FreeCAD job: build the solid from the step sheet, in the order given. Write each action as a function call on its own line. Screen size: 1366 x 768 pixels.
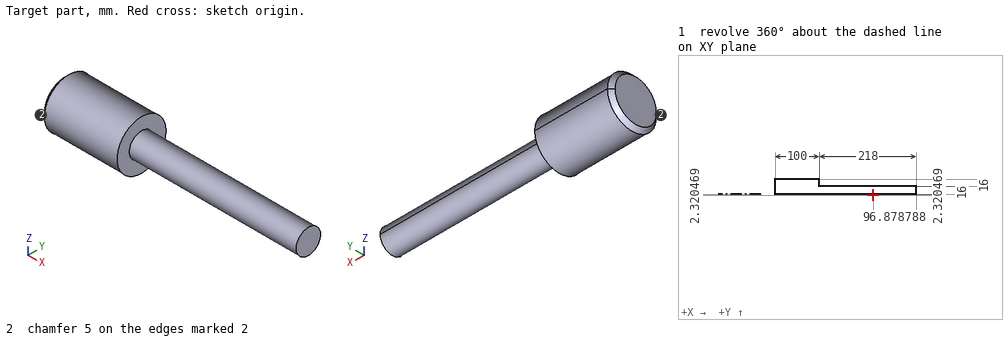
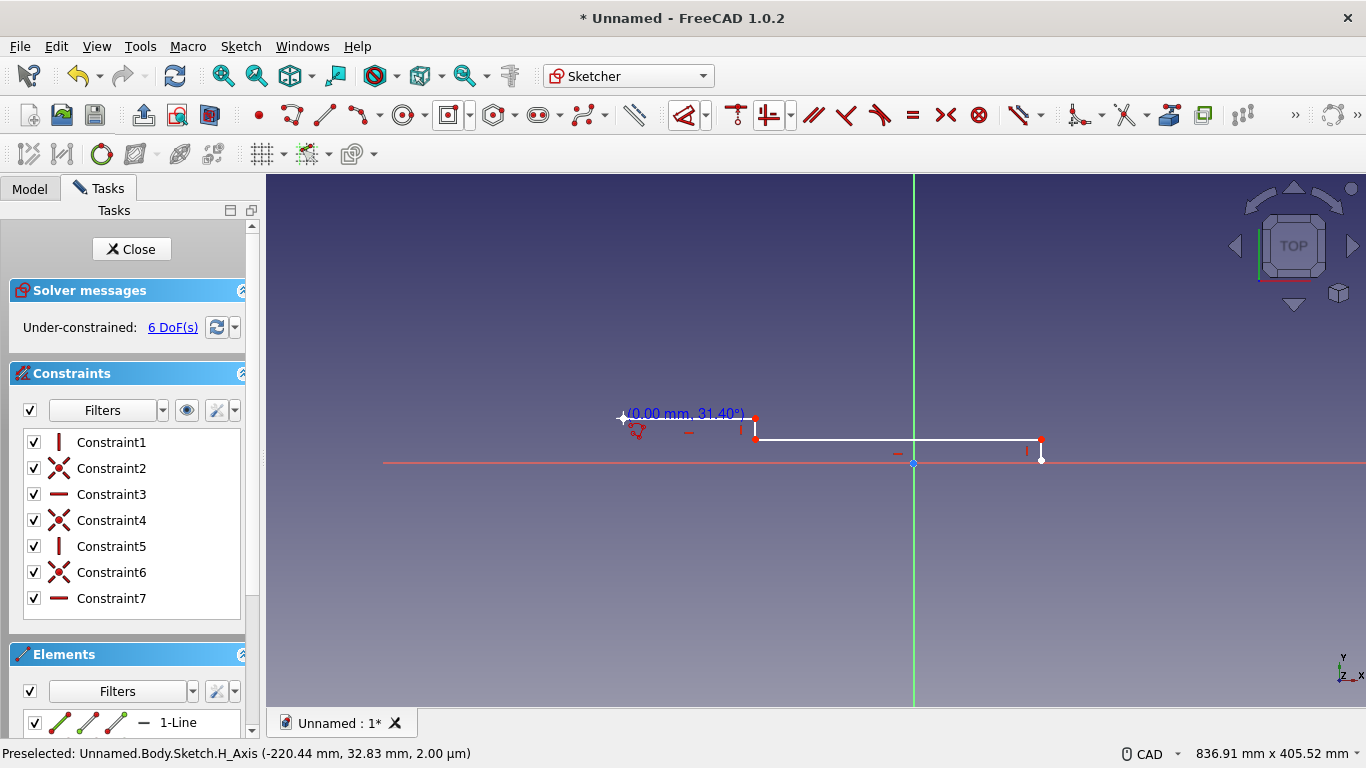
scroll(623, 460, up, 9)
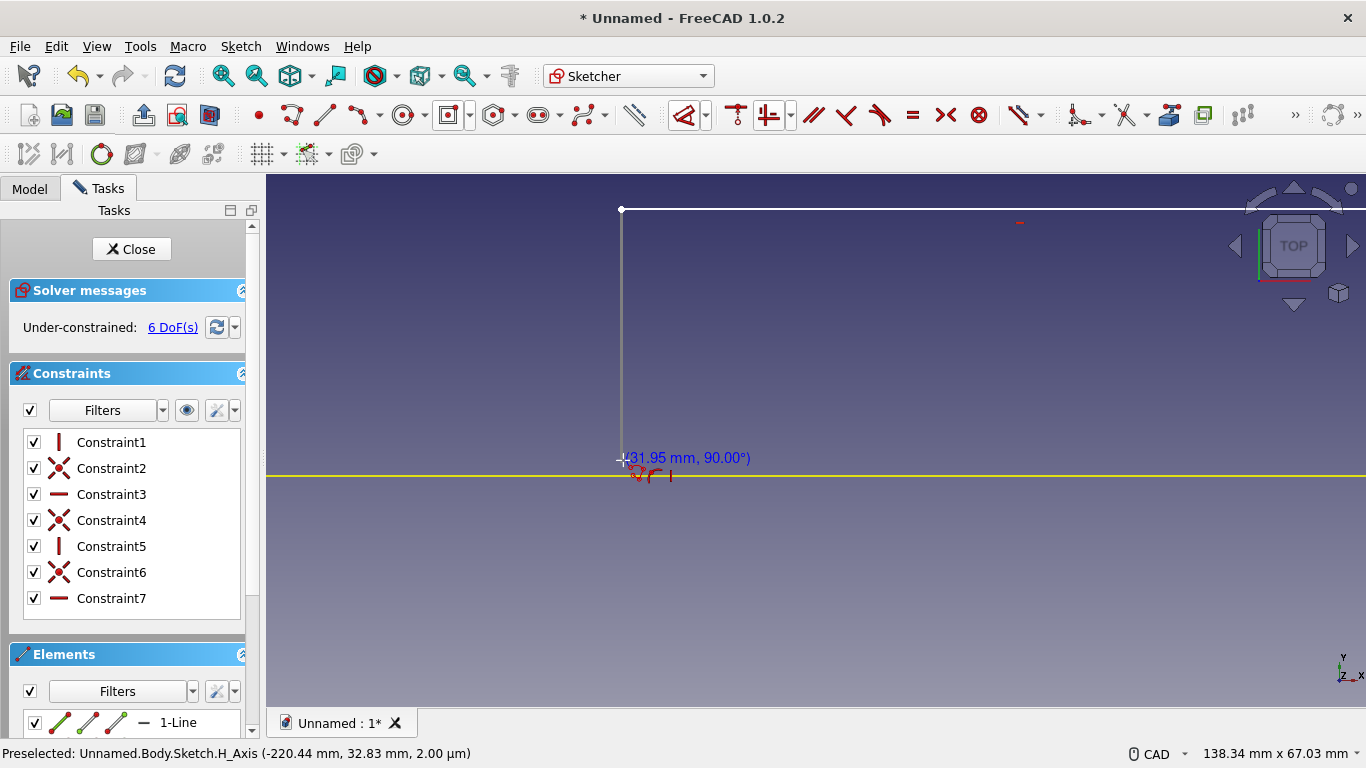
click(621, 458)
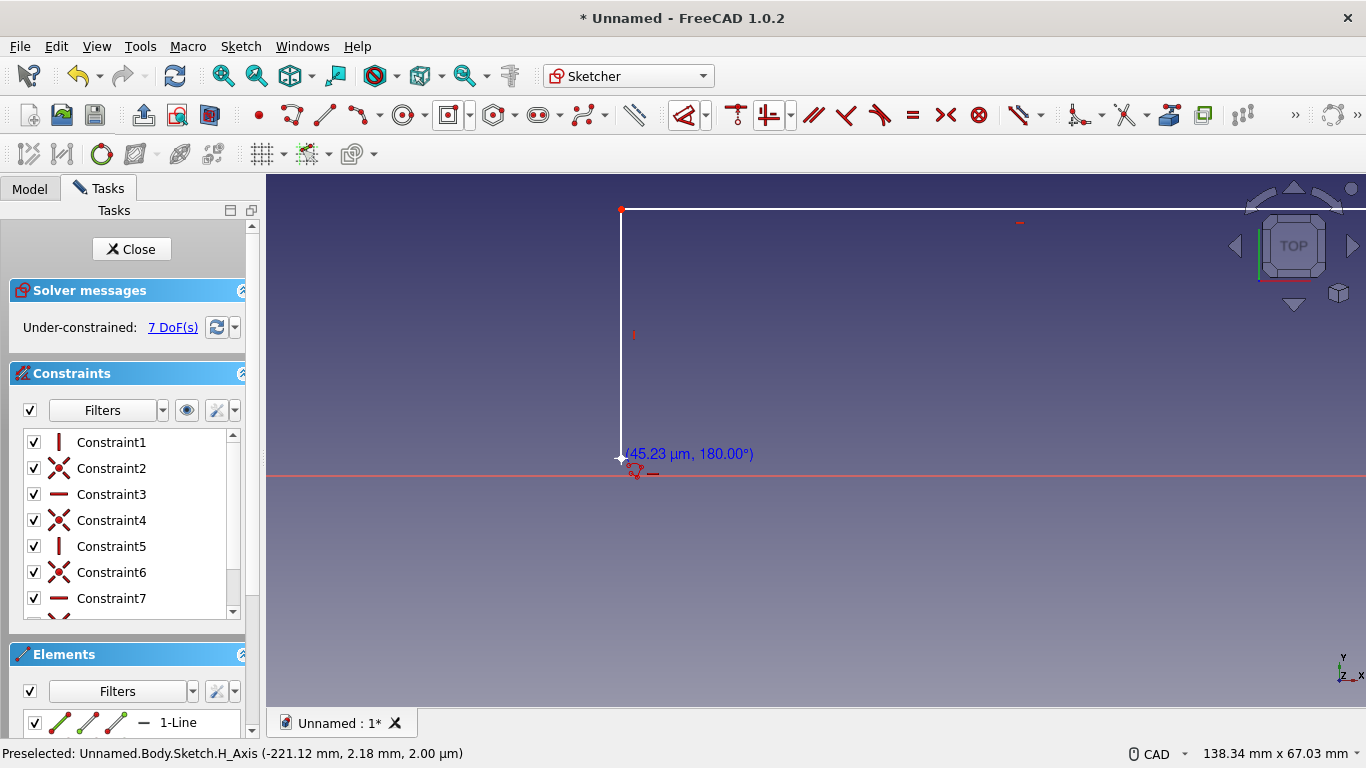
scroll(622, 460, down, 9)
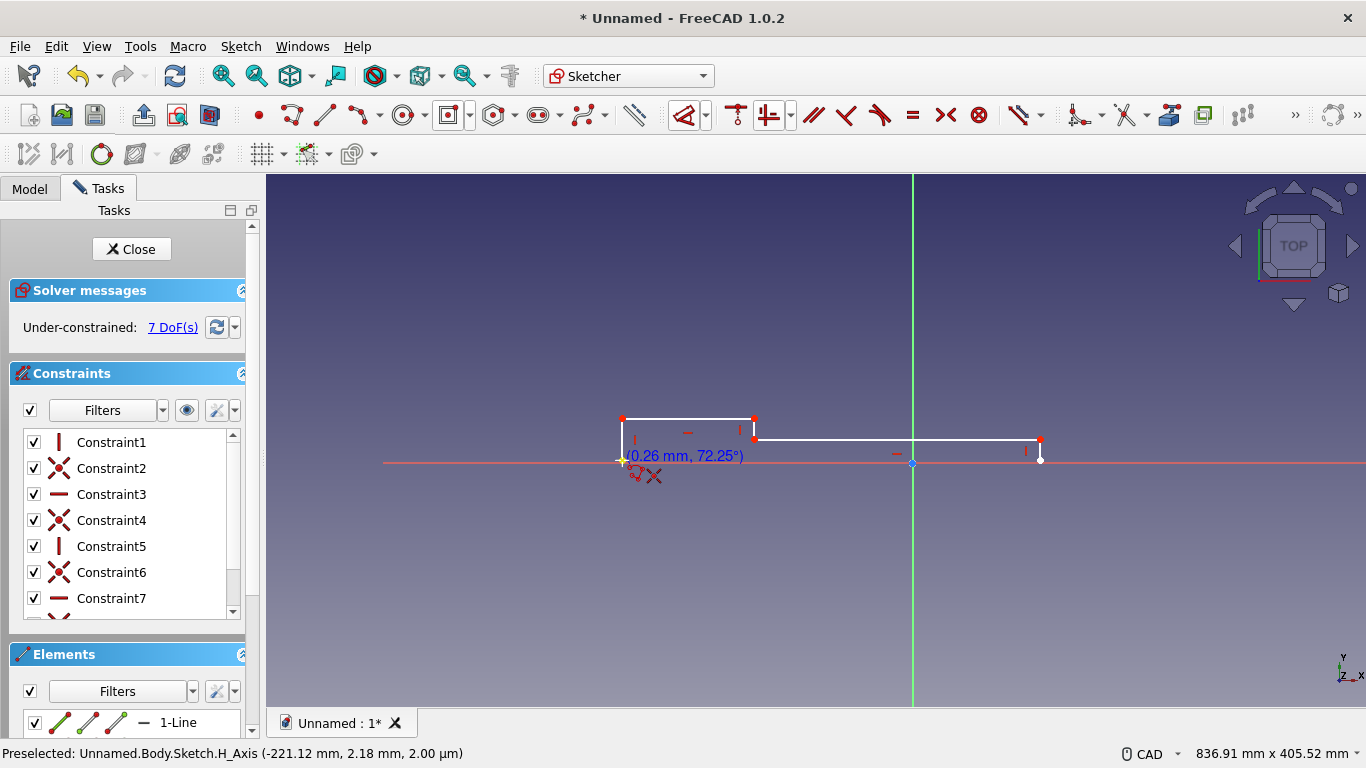
scroll(1040, 460, up, 9)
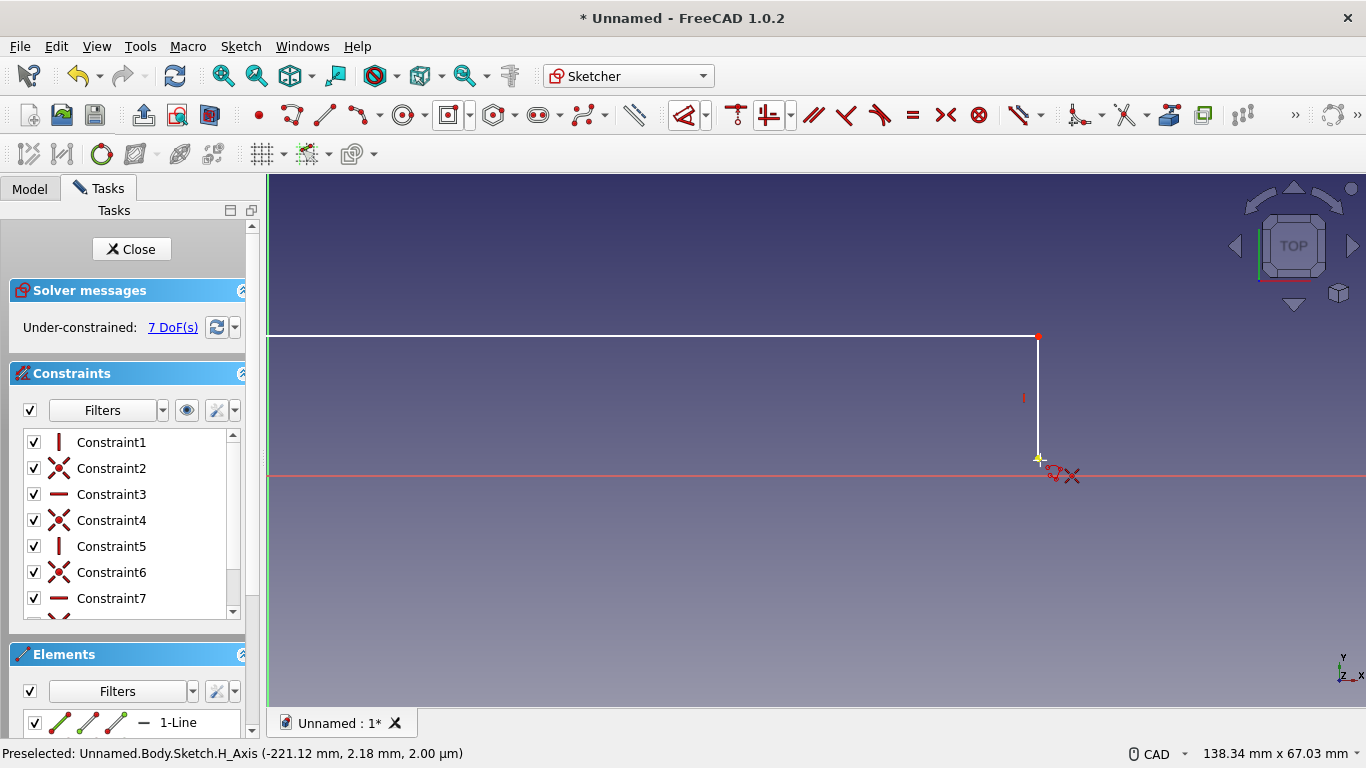
click(1038, 459)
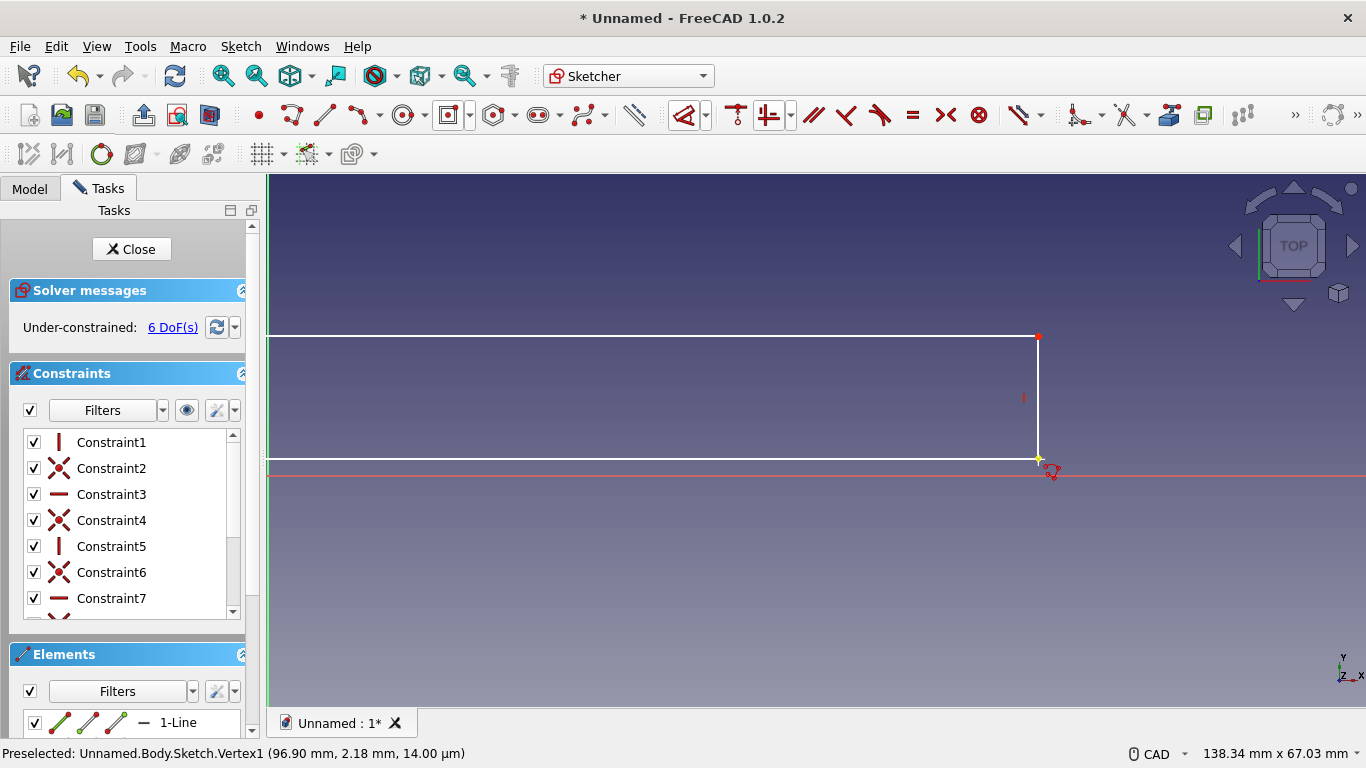
click(325, 116)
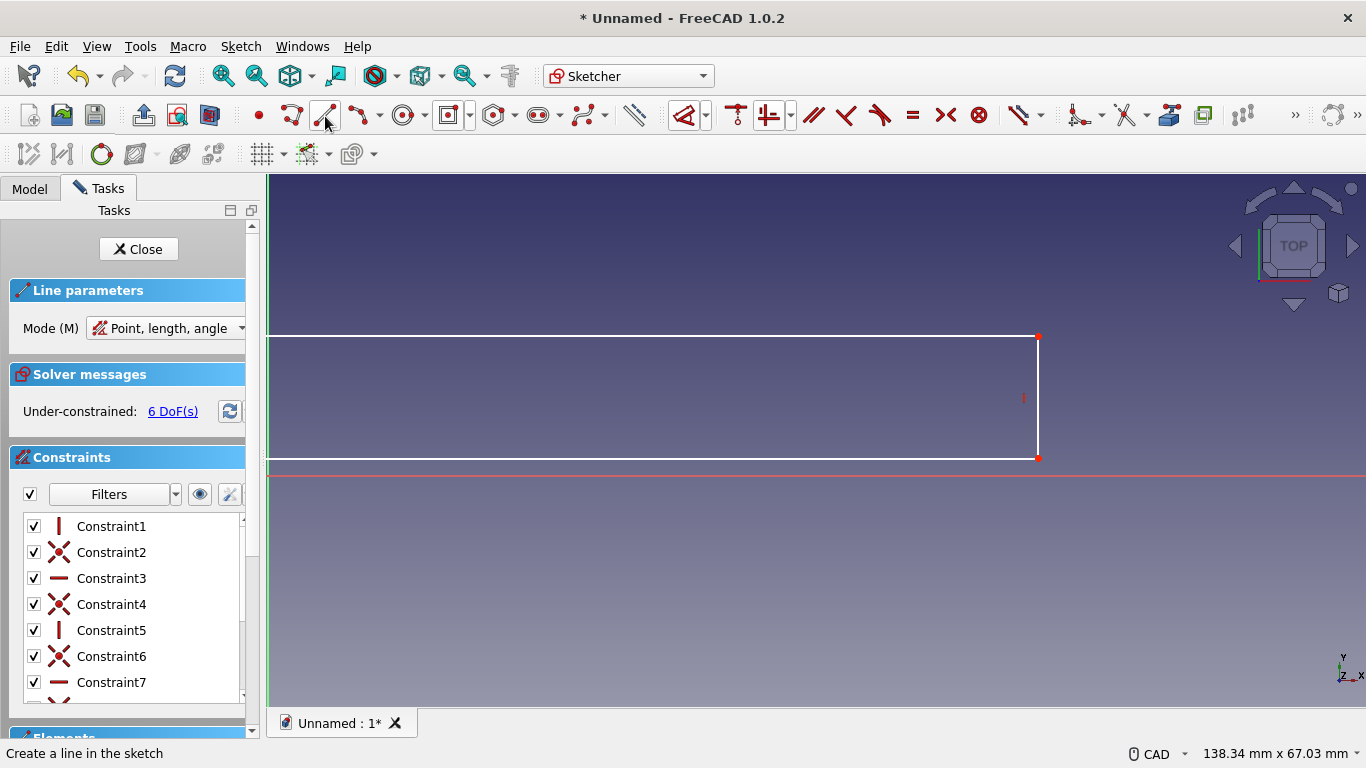
scroll(1041, 460, down, 9)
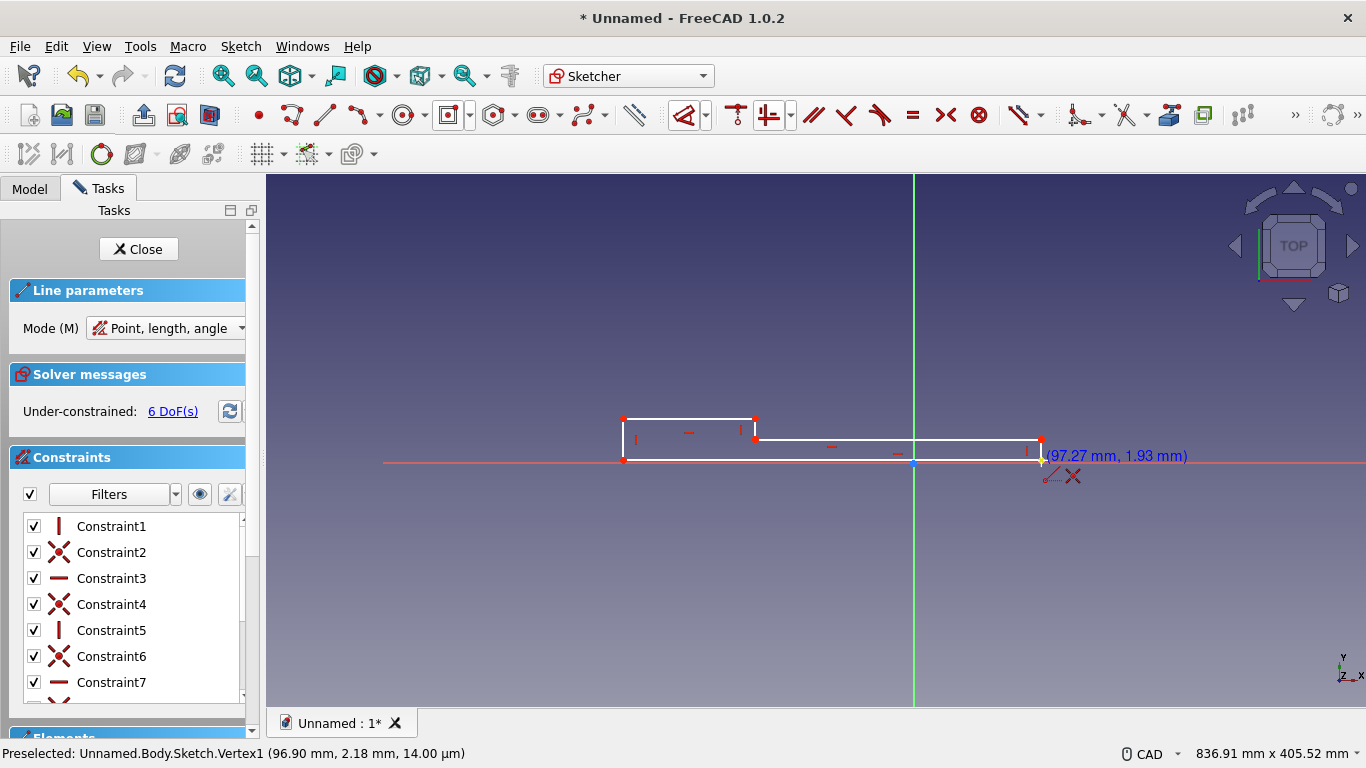
scroll(581, 460, up, 9)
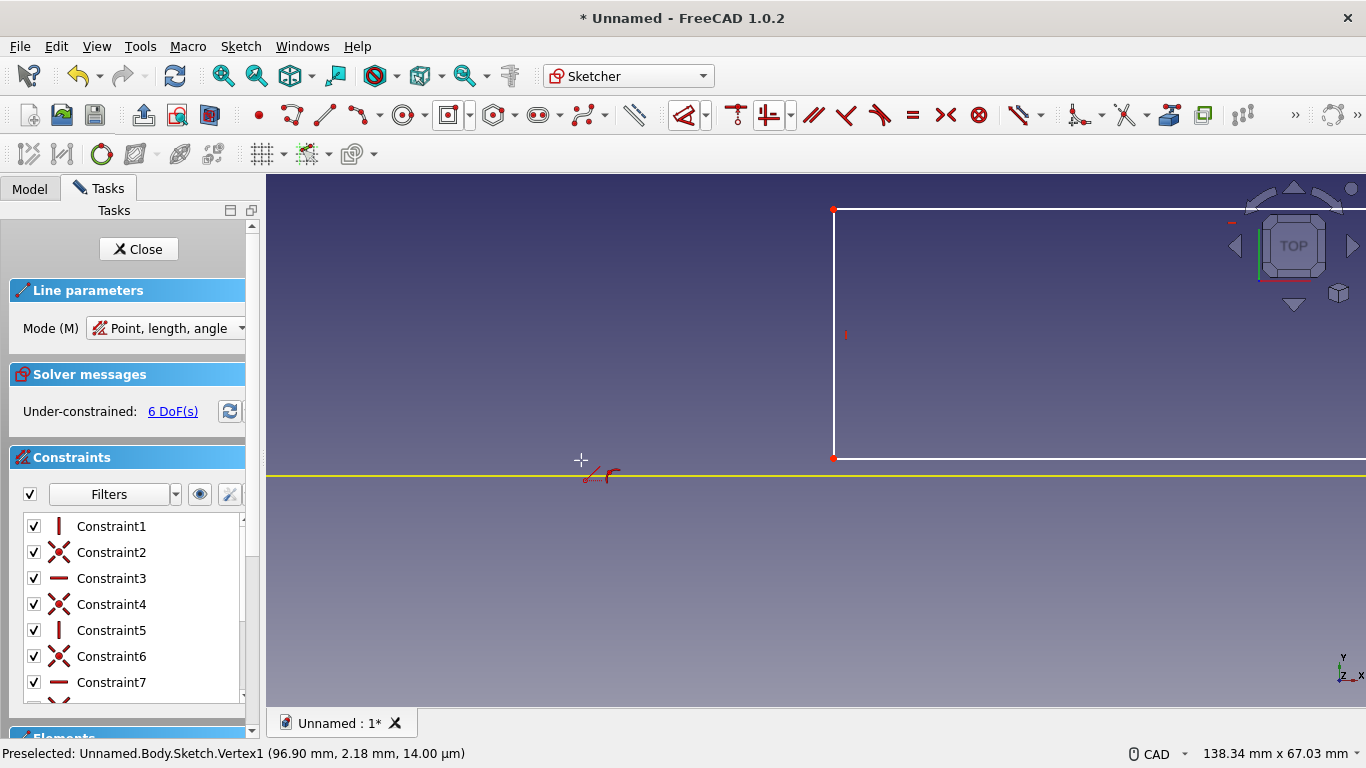
click(581, 458)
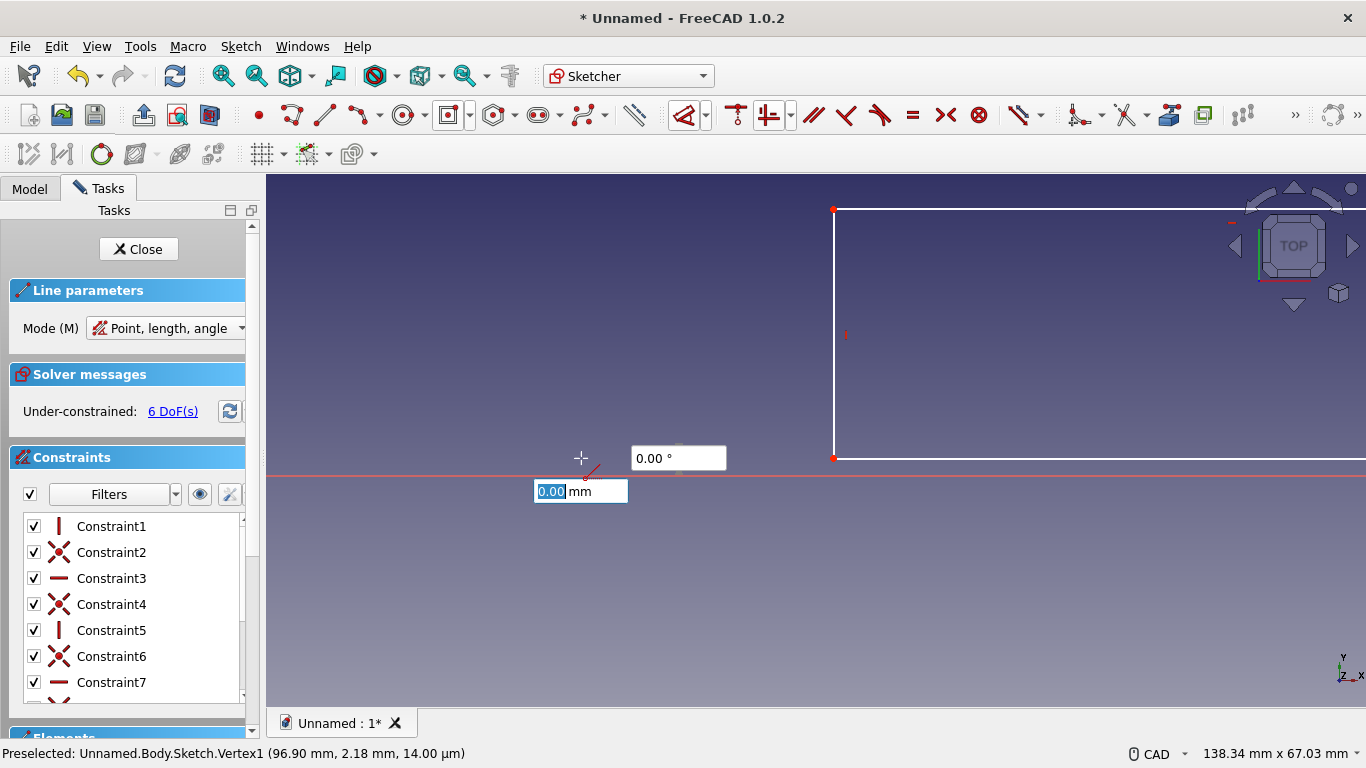
scroll(580, 460, down, 9)